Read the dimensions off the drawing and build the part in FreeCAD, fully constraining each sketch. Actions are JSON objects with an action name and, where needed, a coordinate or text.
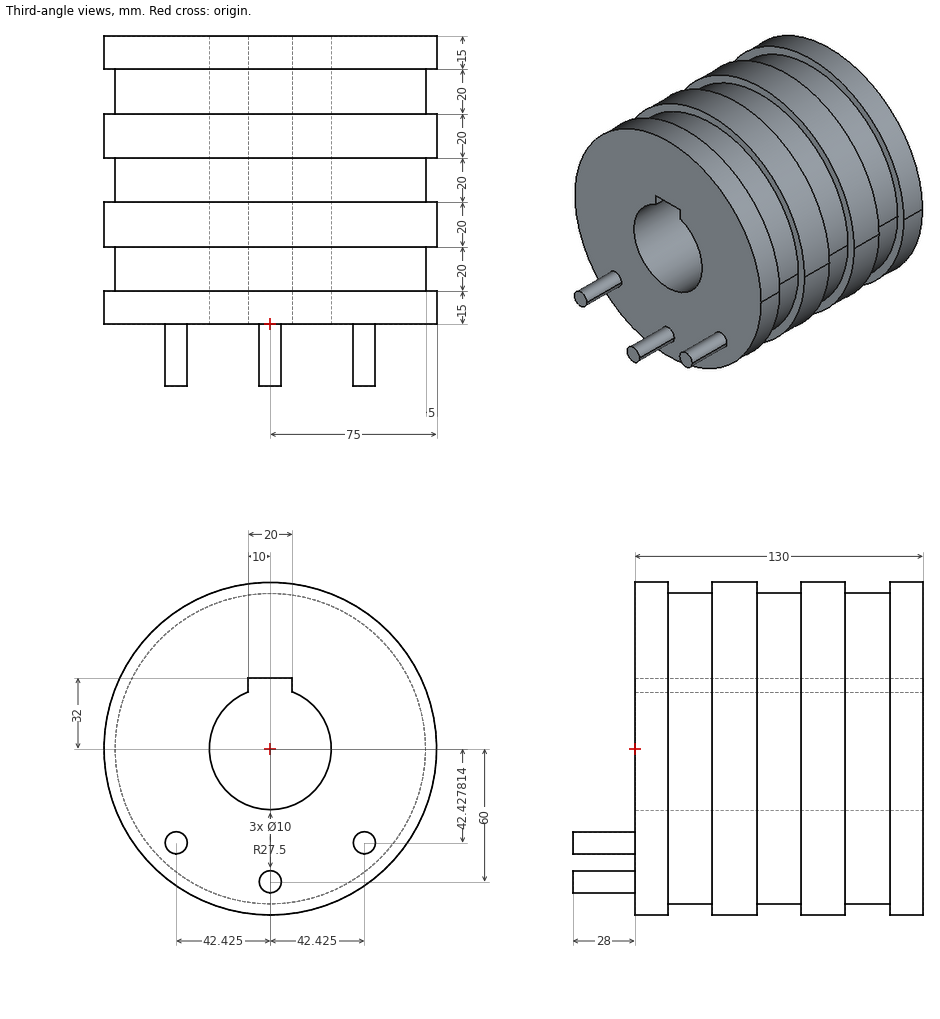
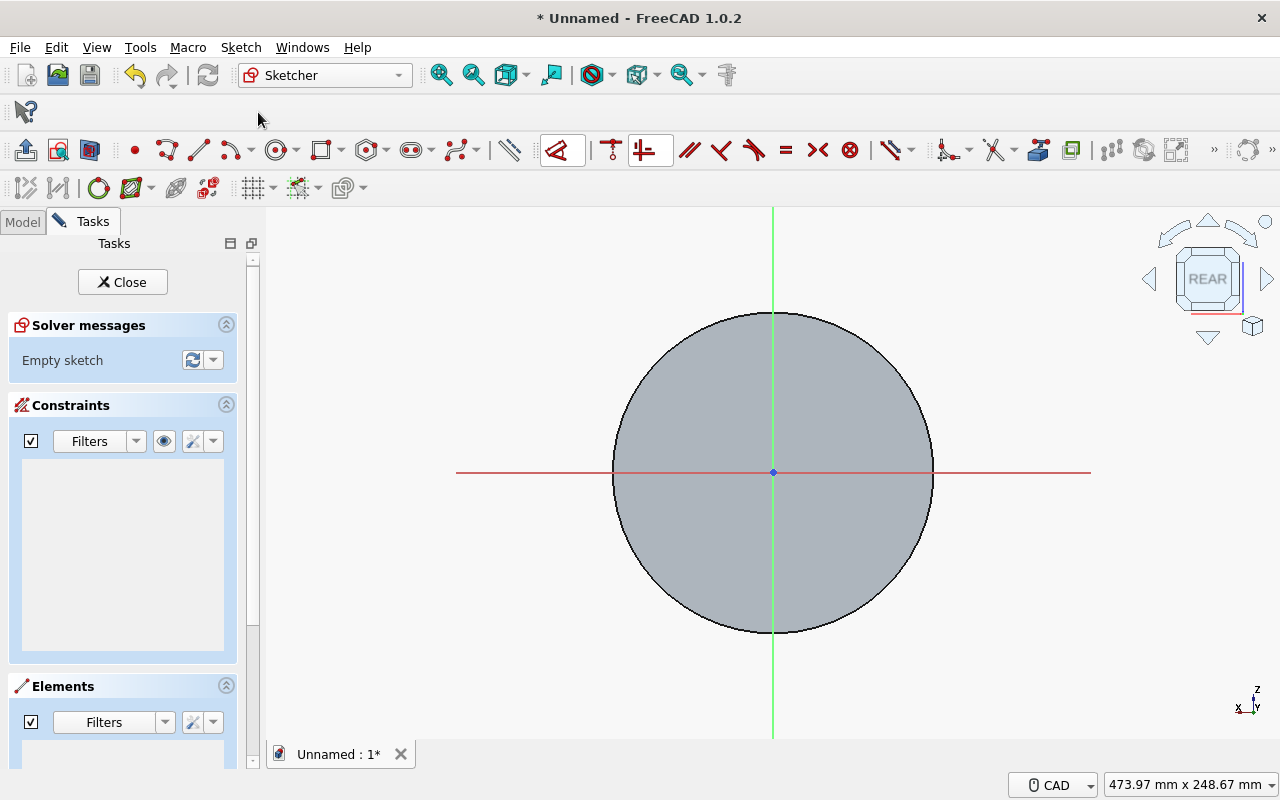
{"action": "scroll", "coordinate": [813, 465], "scroll_direction": "up", "scroll_amount": 5}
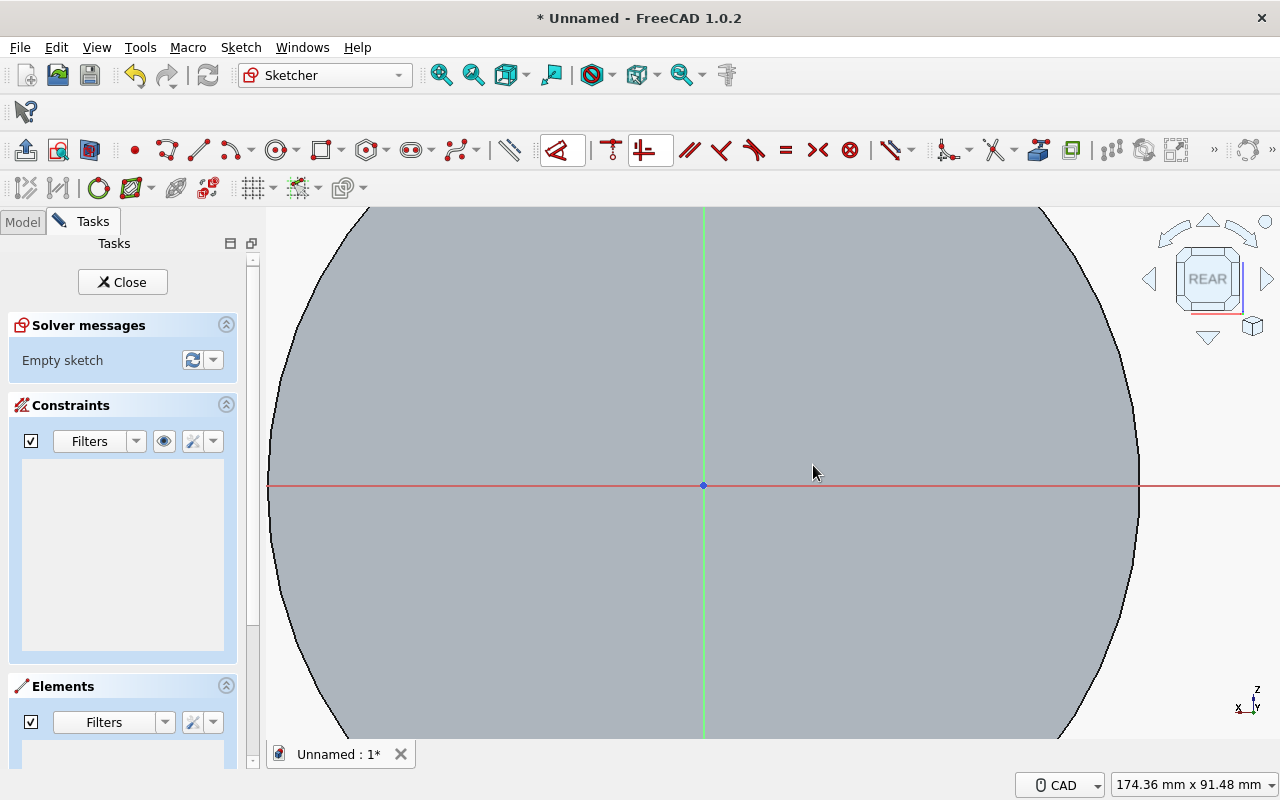
{"action": "key", "text": "g m"}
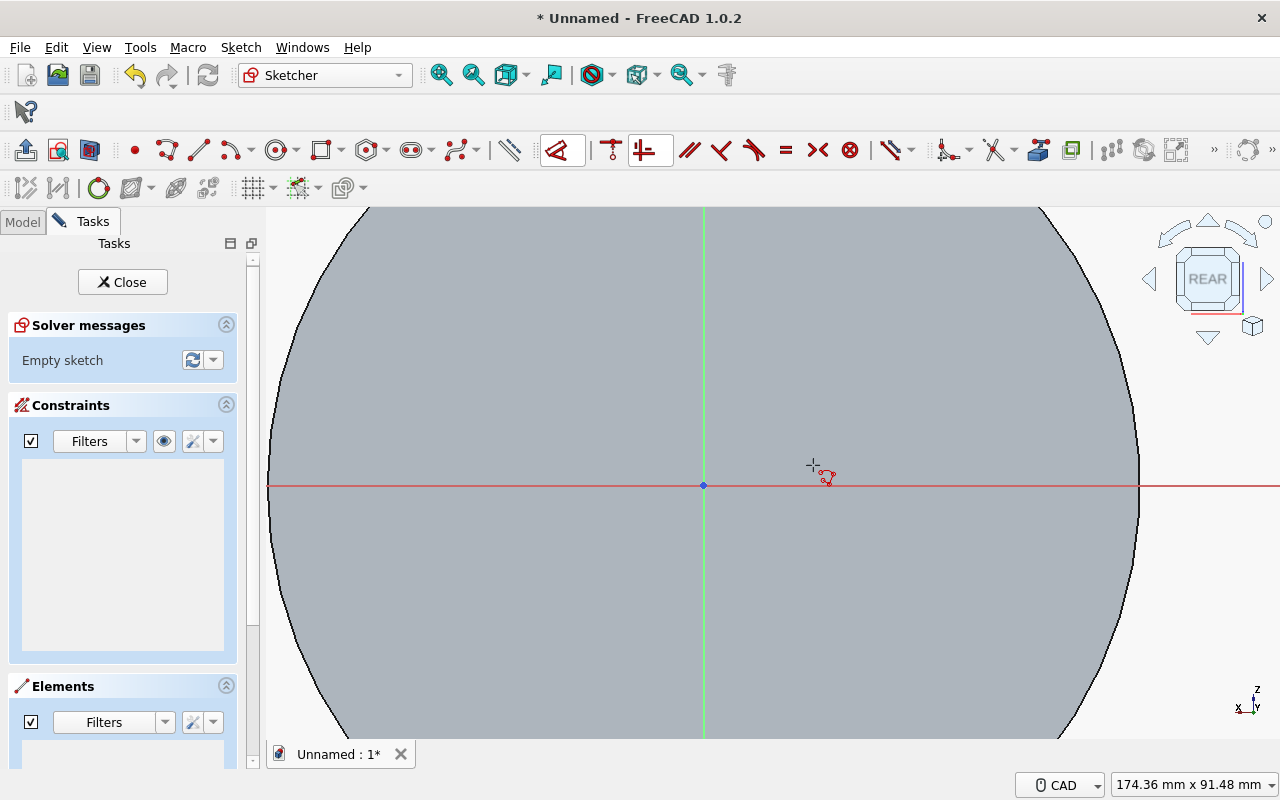
{"action": "left_click", "coordinate": [762, 337]}
{"action": "left_click", "coordinate": [762, 300]}
{"action": "left_click", "coordinate": [646, 300]}
{"action": "left_click", "coordinate": [646, 337]}
{"action": "right_click", "coordinate": [646, 337]}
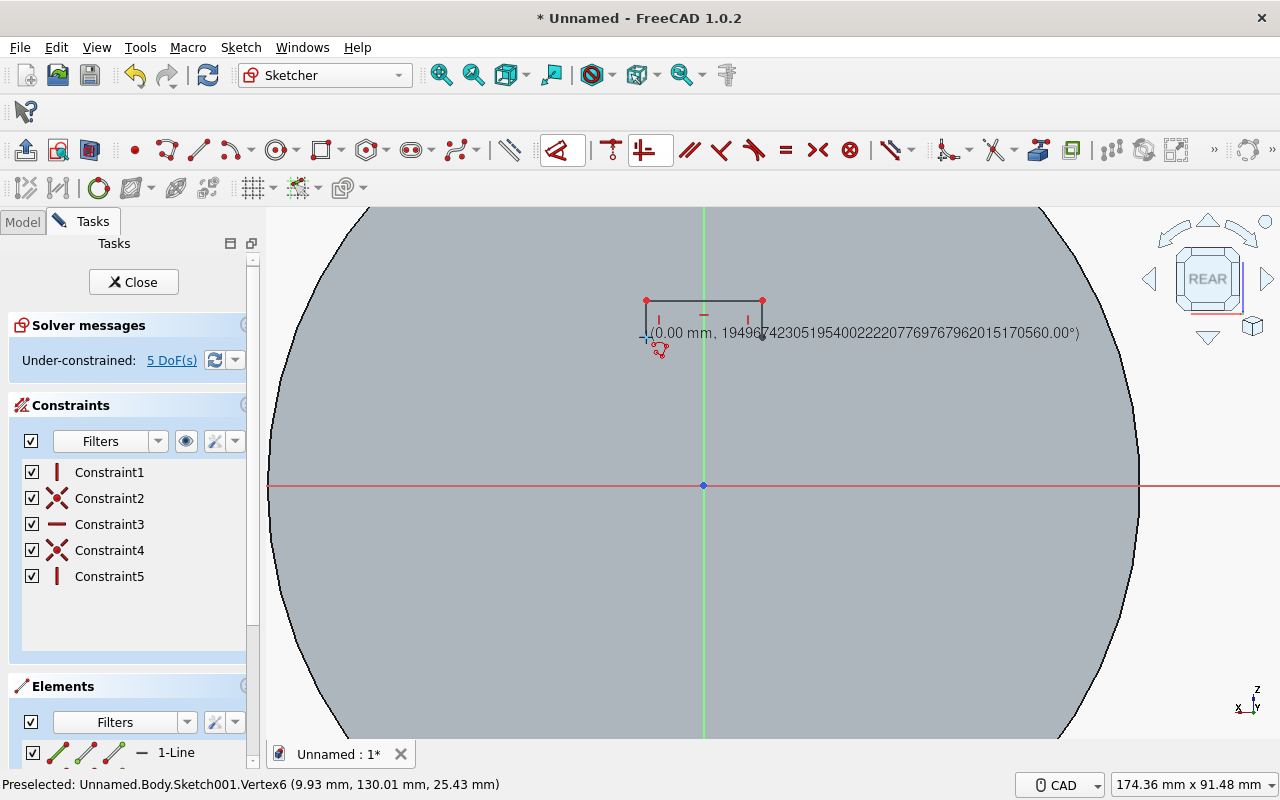
{"action": "left_click", "coordinate": [254, 150]}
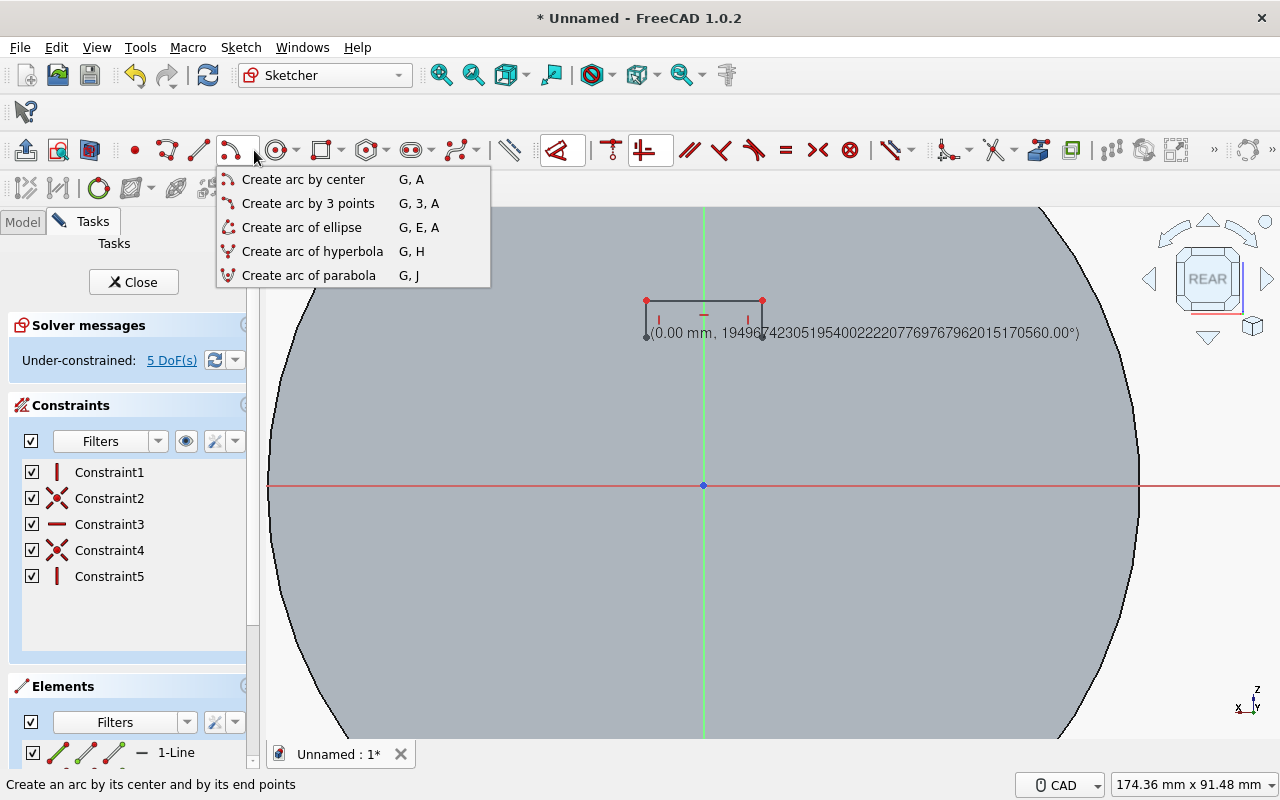
{"action": "left_click", "coordinate": [354, 203]}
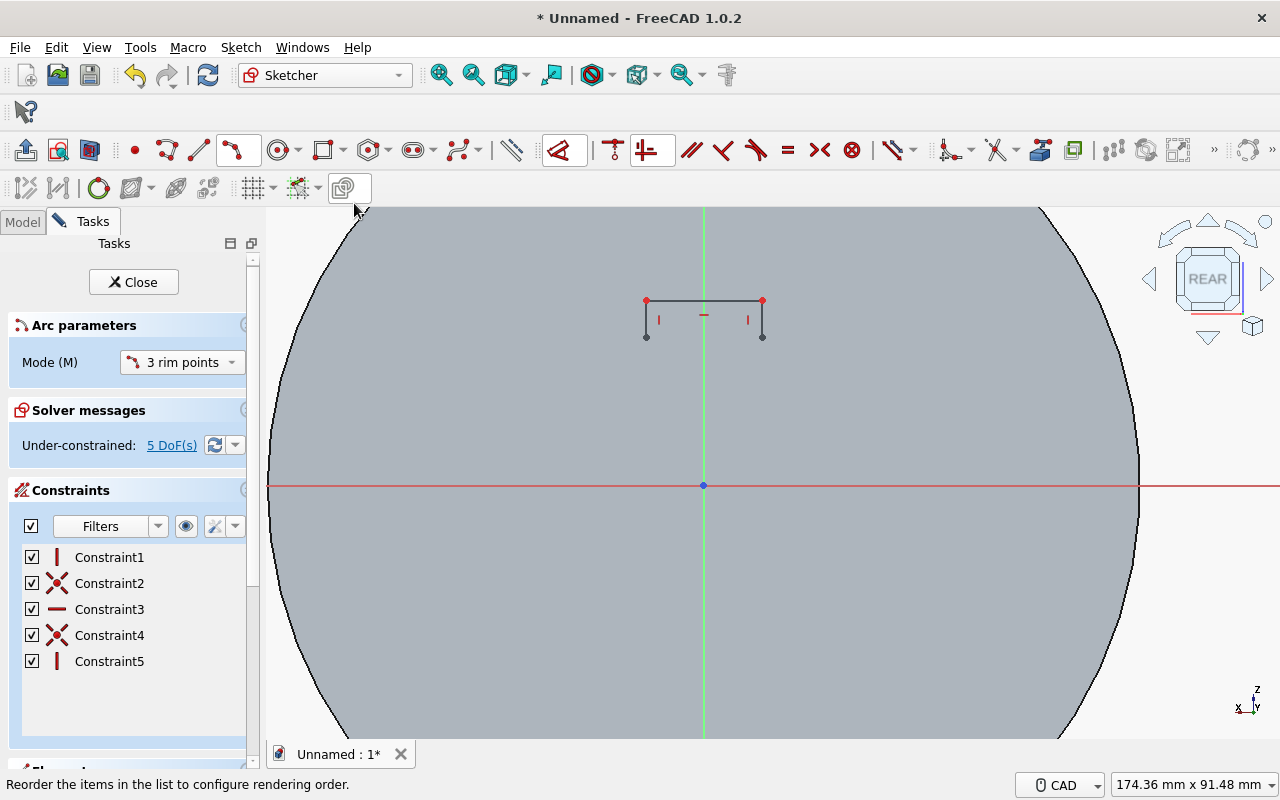
{"action": "left_click", "coordinate": [646, 338]}
{"action": "left_click", "coordinate": [762, 338]}
{"action": "left_click", "coordinate": [620, 622]}
{"action": "key", "text": "Escape"}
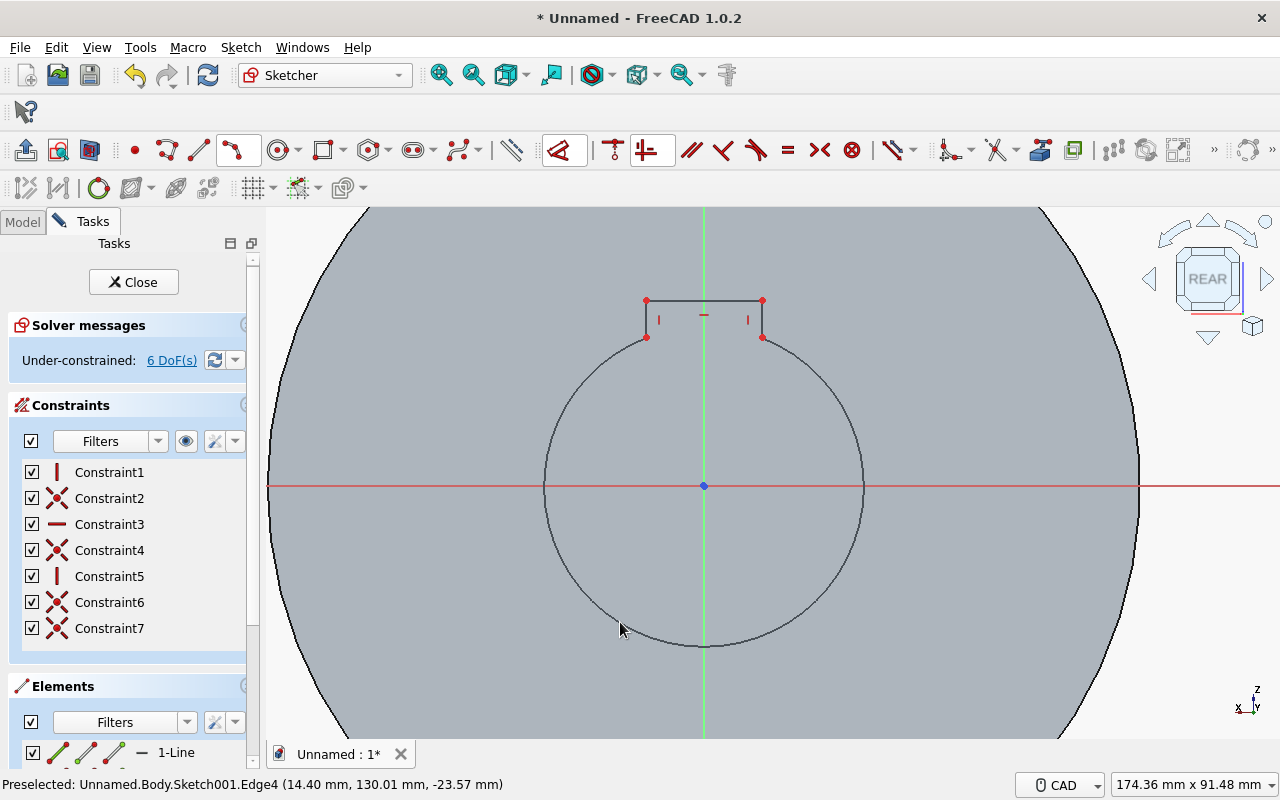
{"action": "left_click_drag", "start_coordinate": [694, 476], "coordinate": [714, 497]}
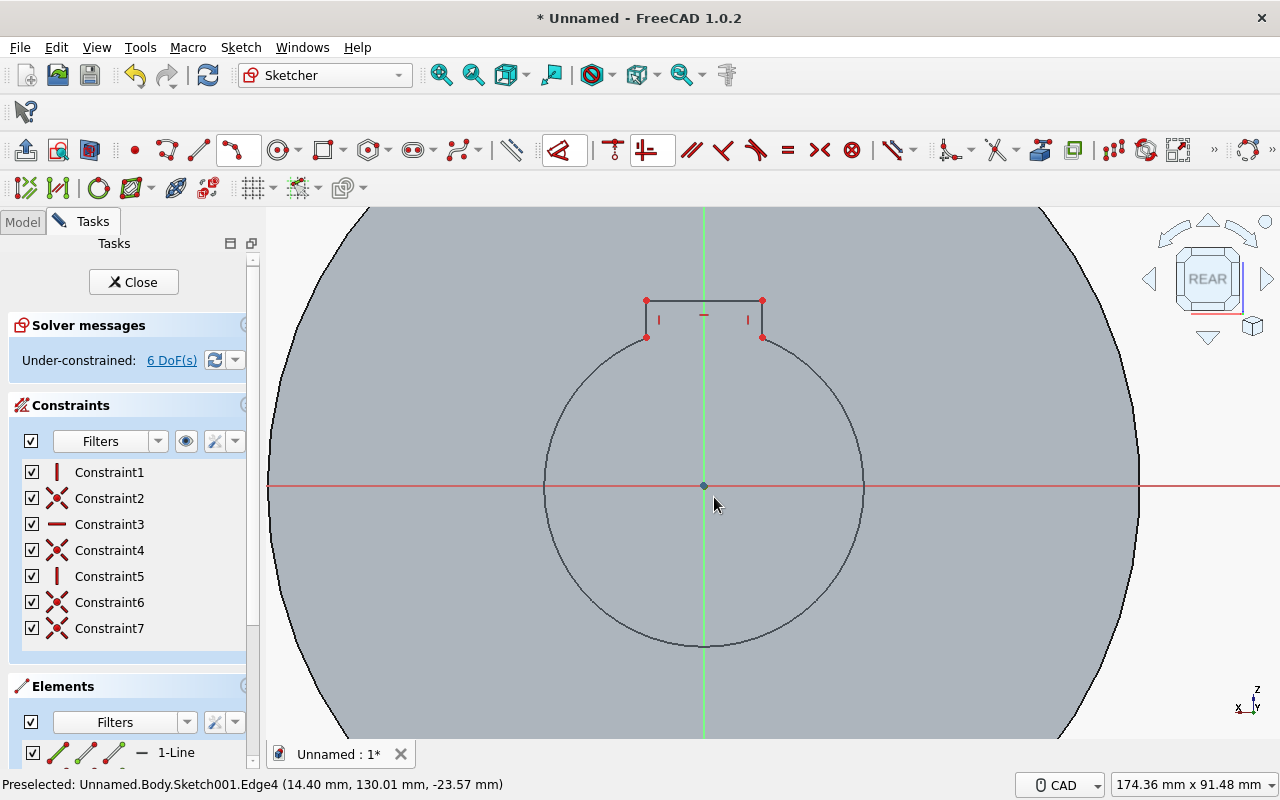
{"action": "left_click", "coordinate": [614, 150]}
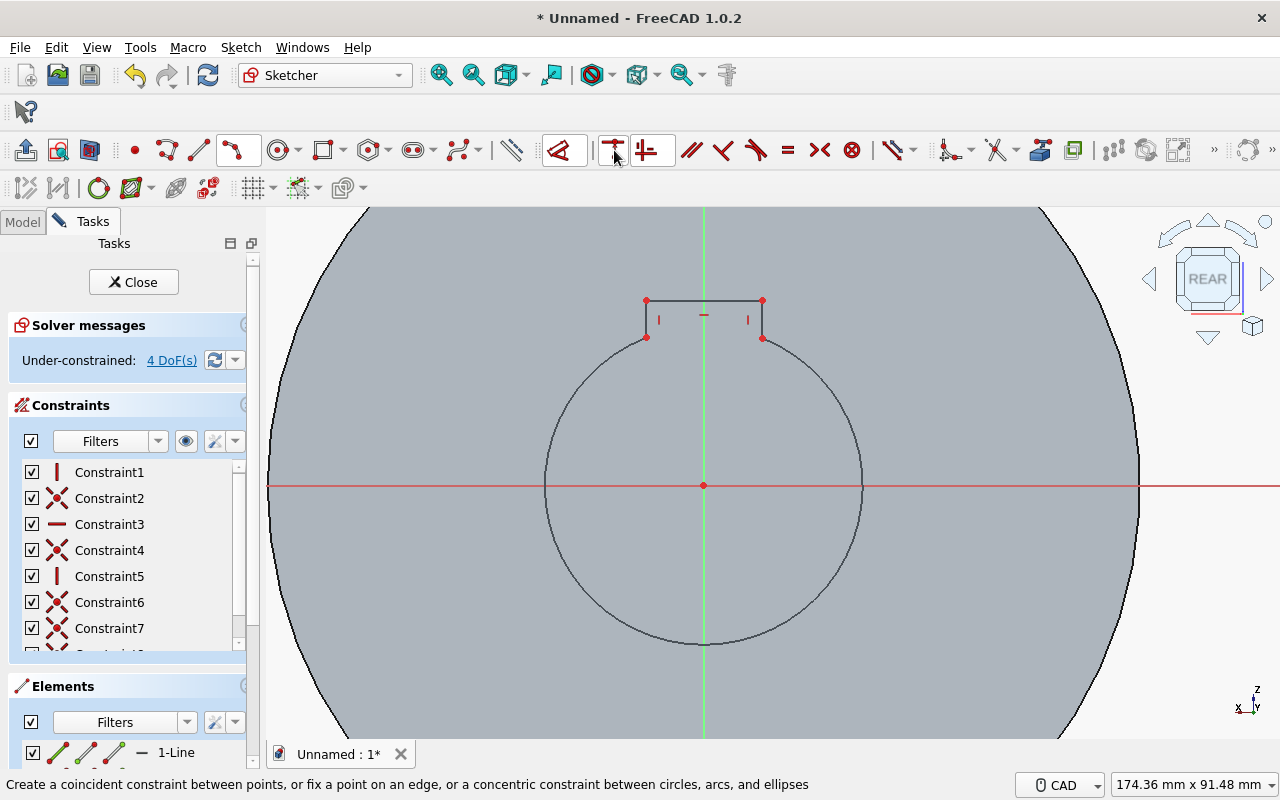
{"action": "left_click", "coordinate": [561, 557]}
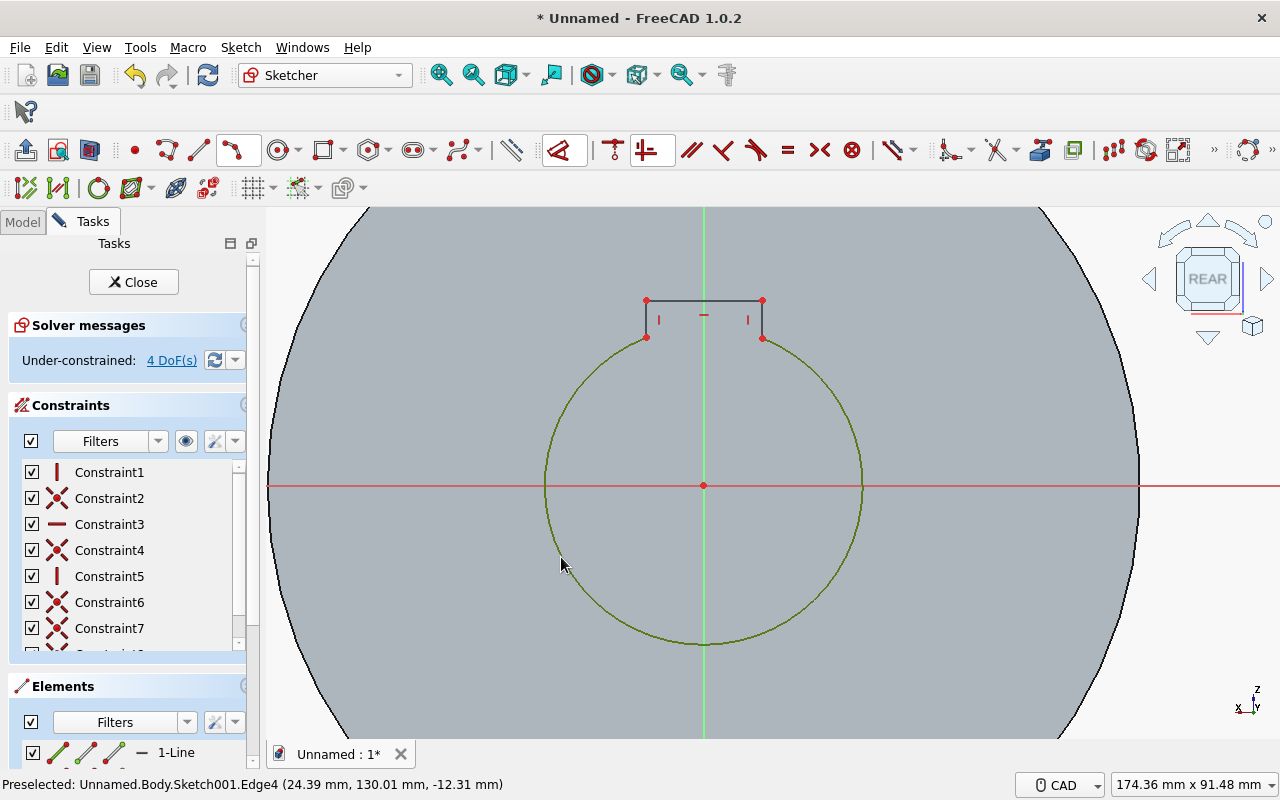
{"action": "key", "text": "k r"}